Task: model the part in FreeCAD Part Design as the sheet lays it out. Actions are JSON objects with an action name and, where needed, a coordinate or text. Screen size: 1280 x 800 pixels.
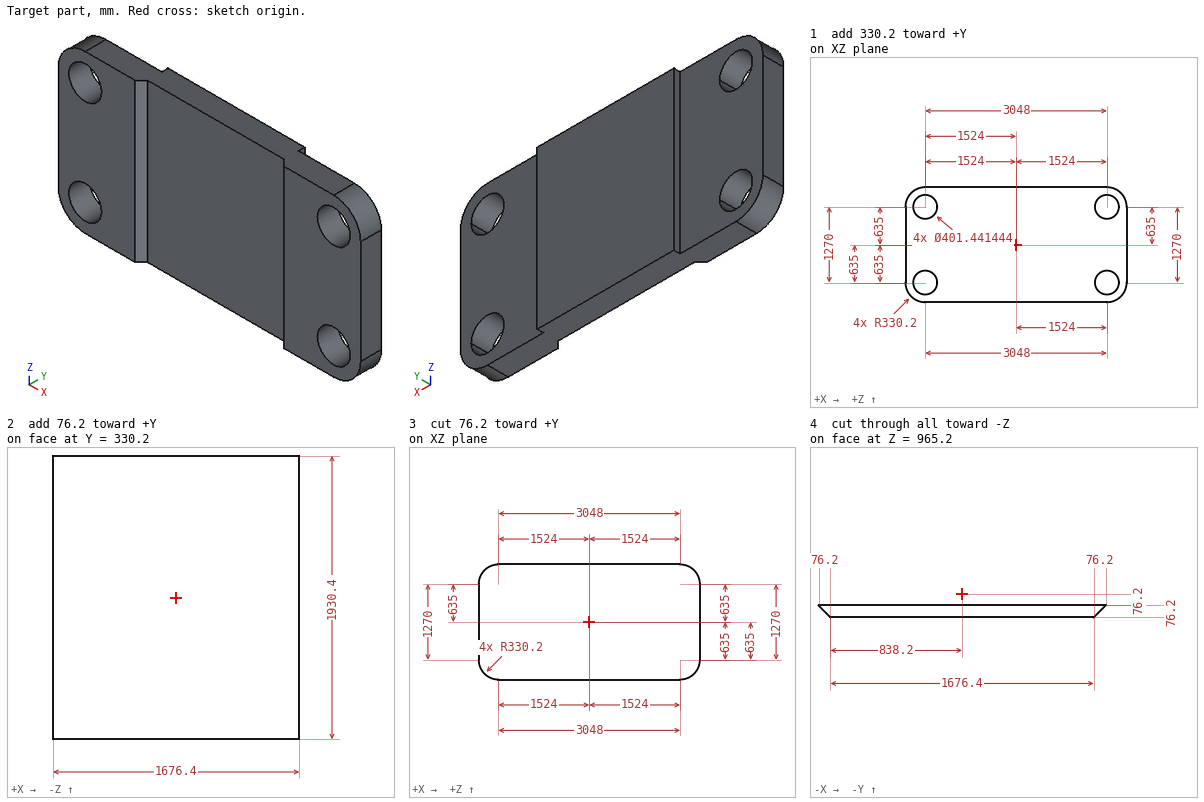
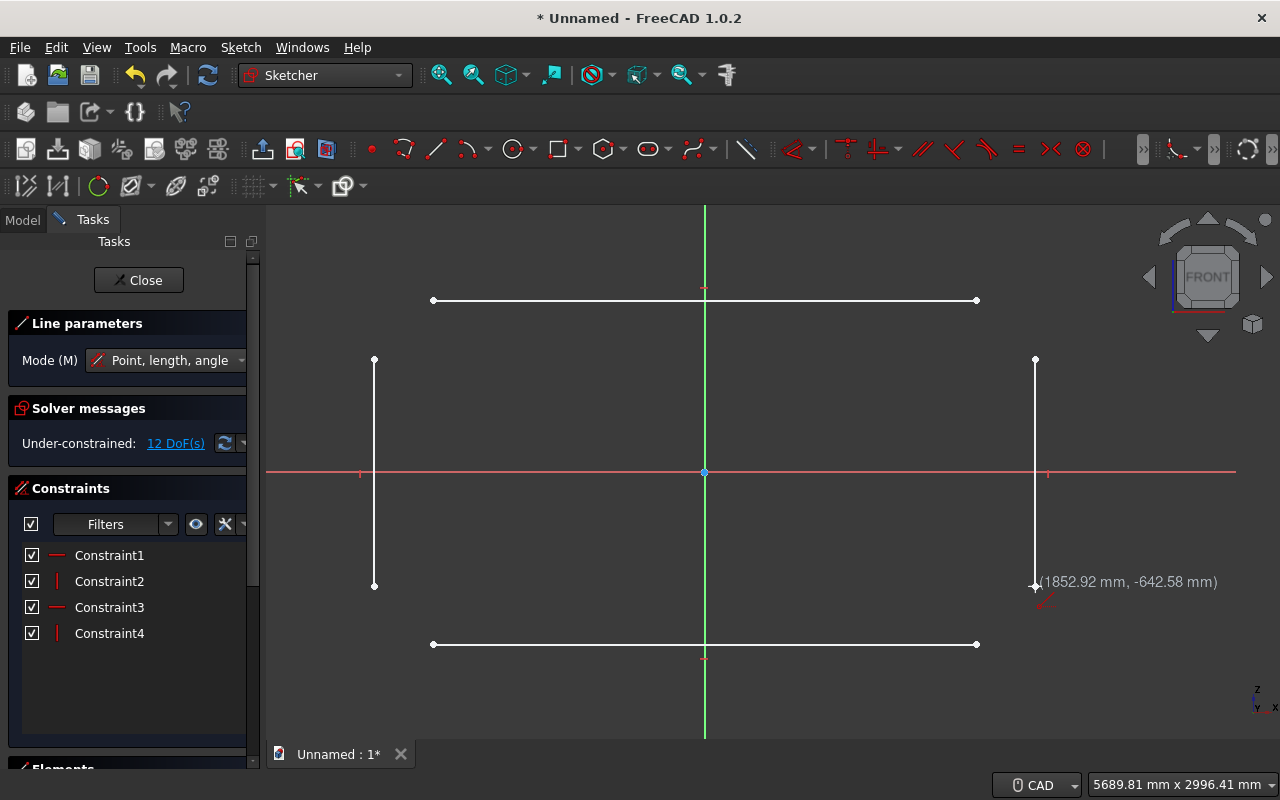
{"action": "key", "text": "g 3 a"}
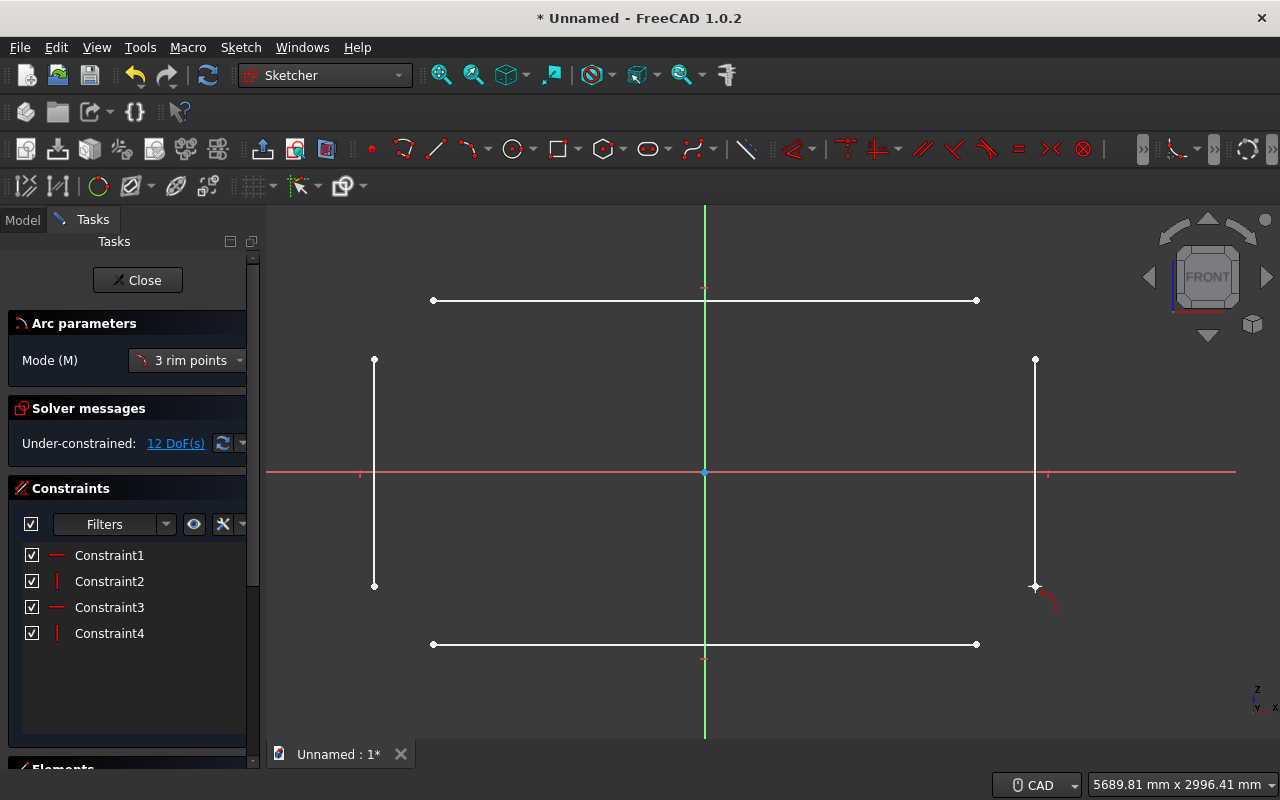
{"action": "left_click", "coordinate": [433, 645]}
{"action": "left_click", "coordinate": [374, 587]}
{"action": "left_click", "coordinate": [392, 627]}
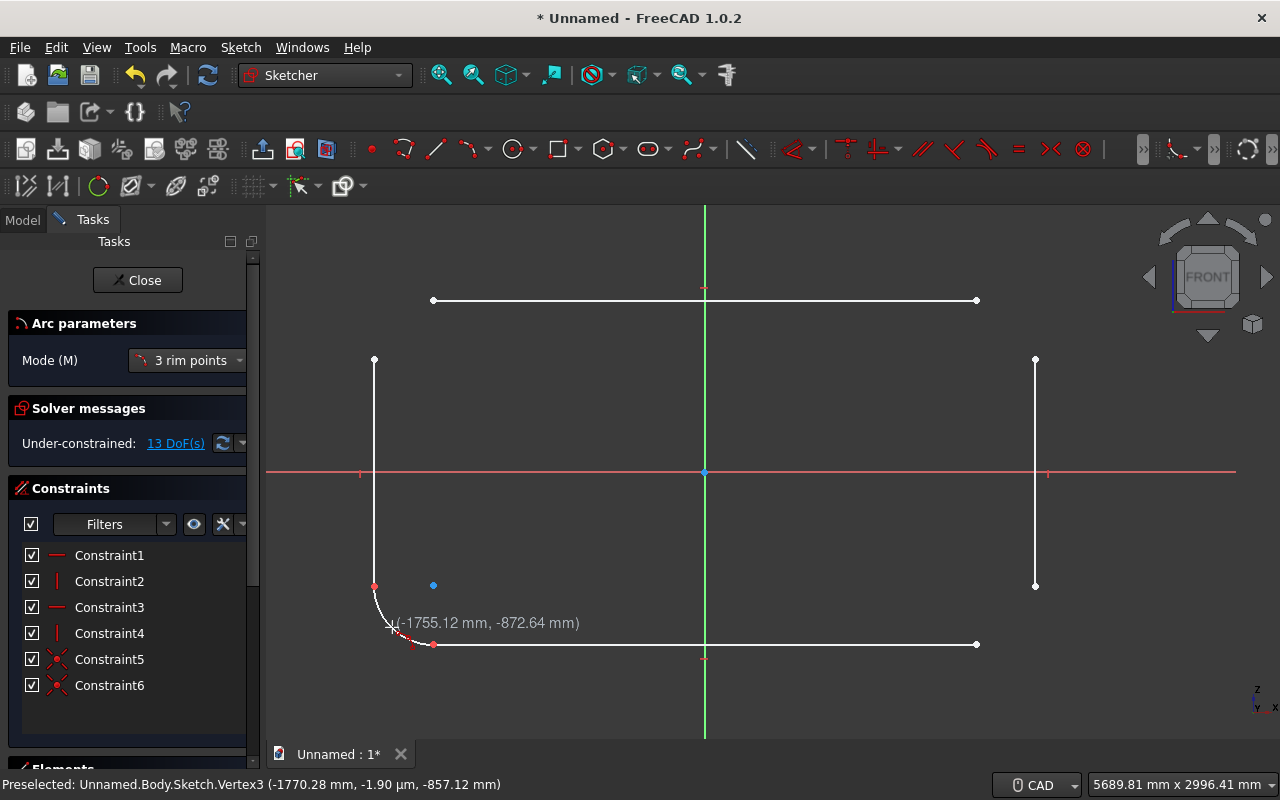
{"action": "left_click", "coordinate": [374, 360]}
{"action": "left_click", "coordinate": [433, 301]}
{"action": "left_click", "coordinate": [392, 318]}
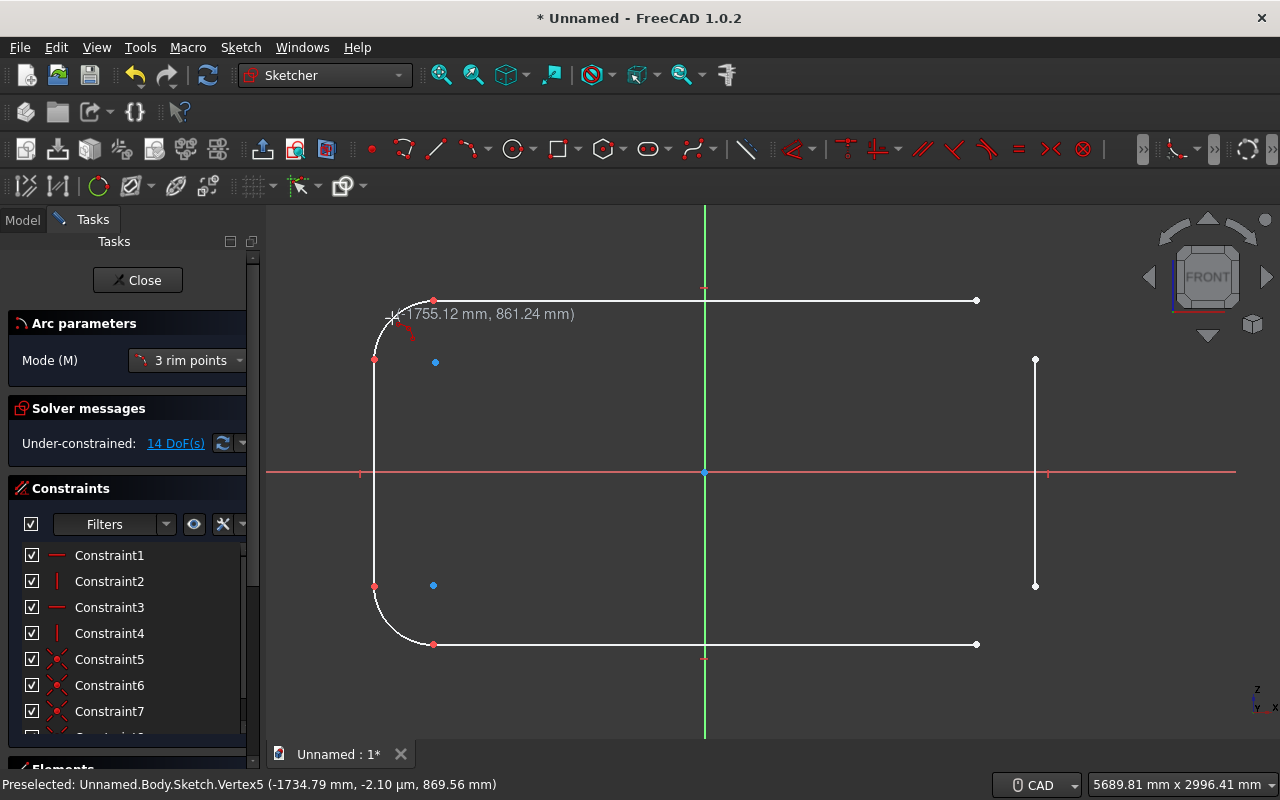
{"action": "left_click", "coordinate": [976, 301]}
{"action": "left_click", "coordinate": [1035, 360]}
{"action": "left_click", "coordinate": [1018, 318]}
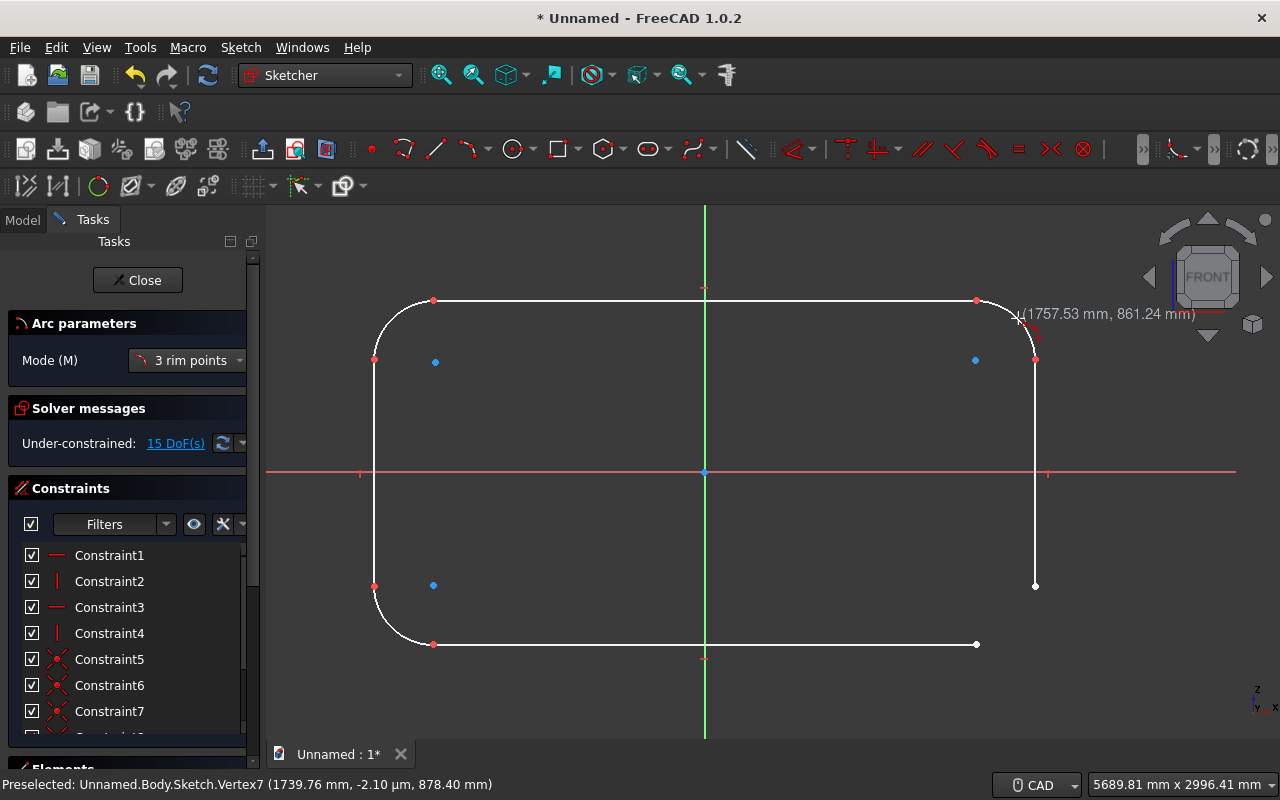
{"action": "left_click", "coordinate": [1035, 587]}
{"action": "left_click", "coordinate": [976, 645]}
{"action": "left_click", "coordinate": [1018, 627]}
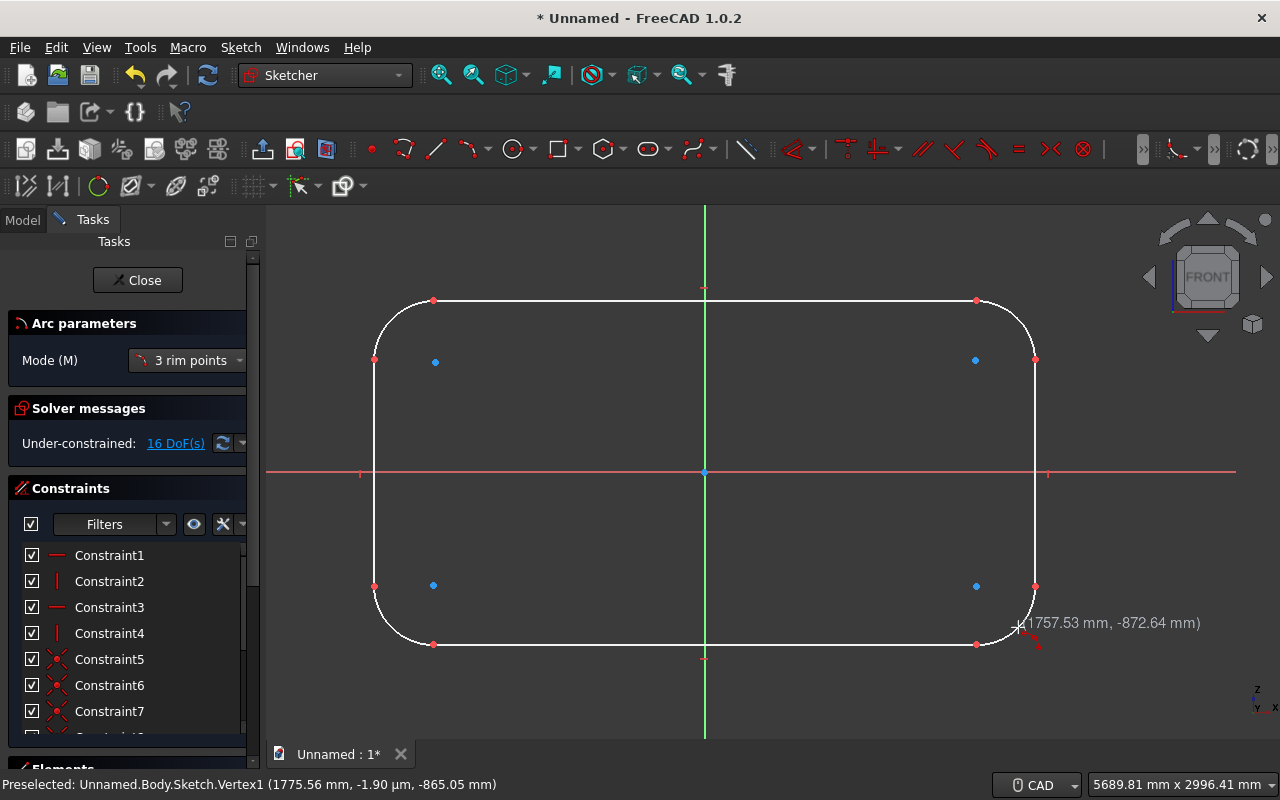
{"action": "key", "text": "g c"}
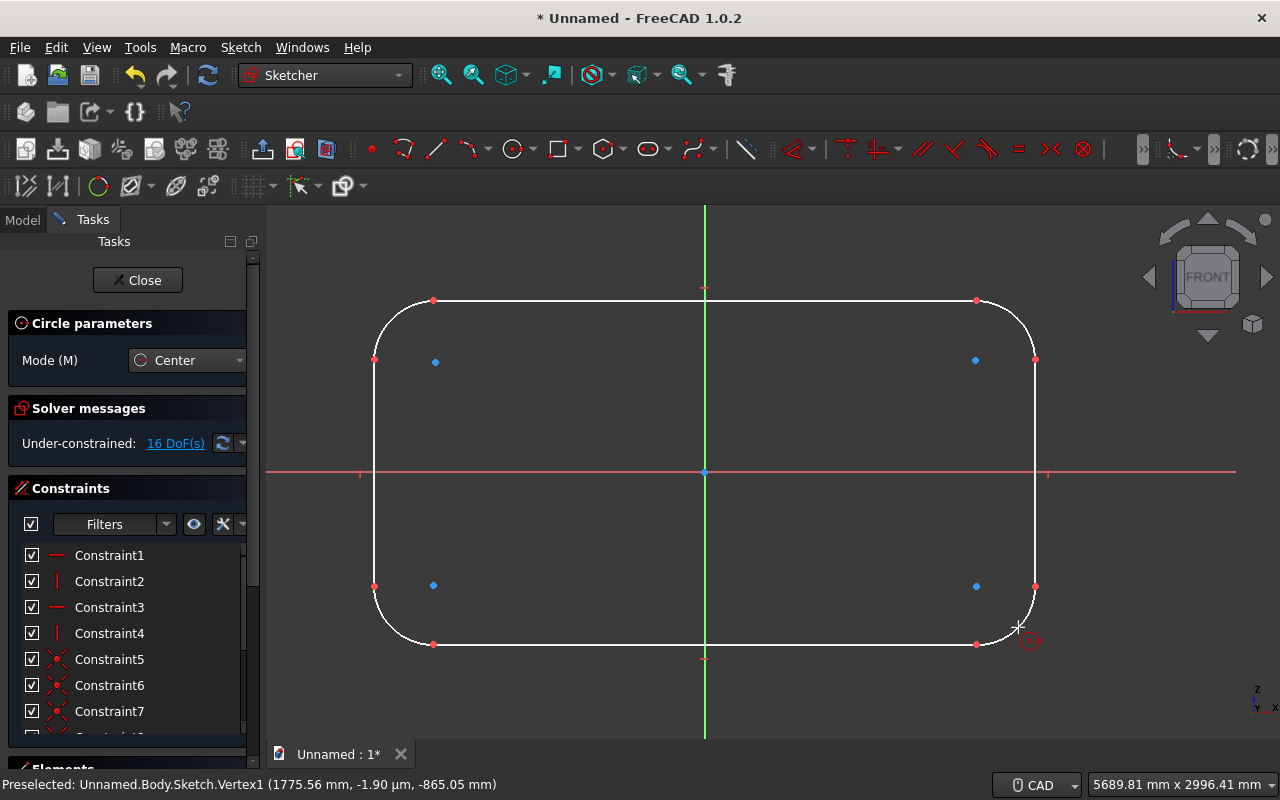
{"action": "left_click", "coordinate": [433, 359]}
{"action": "left_click", "coordinate": [458, 334]}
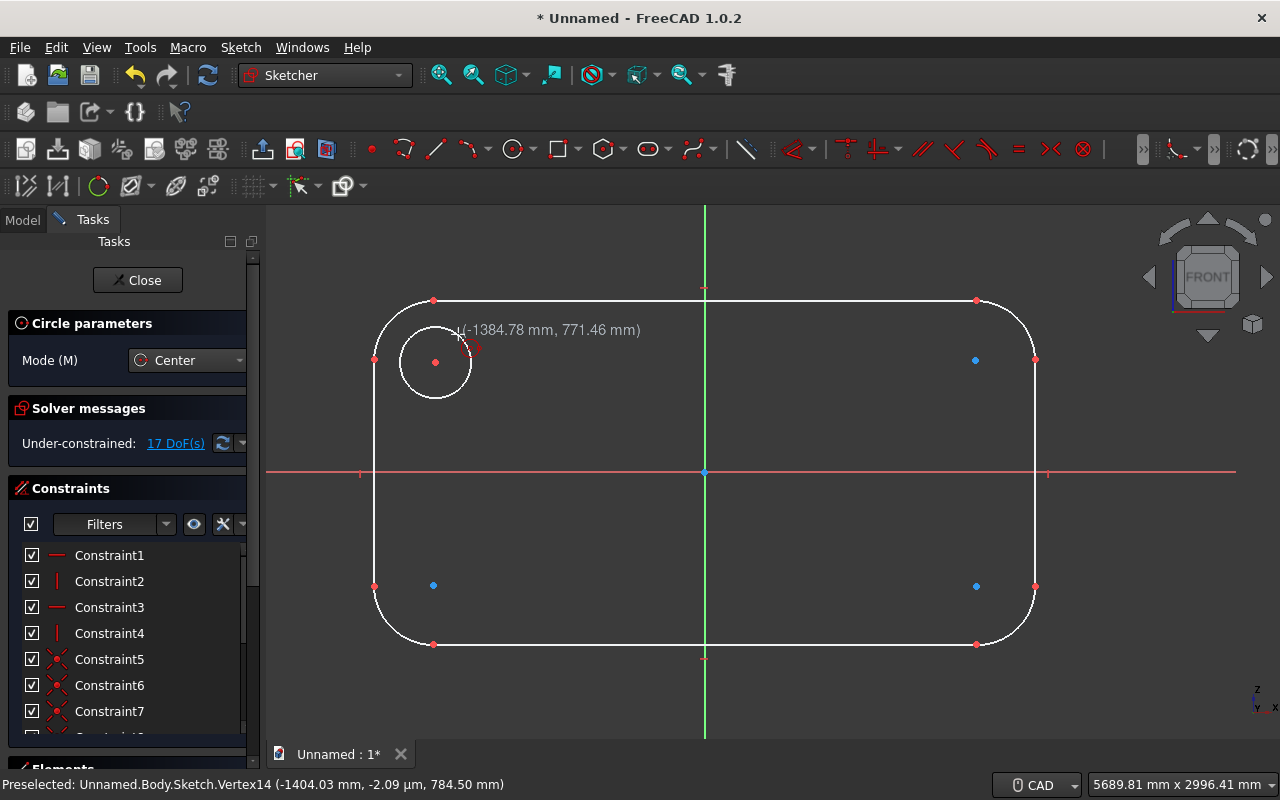
{"action": "left_click", "coordinate": [976, 359]}
{"action": "left_click", "coordinate": [1002, 334]}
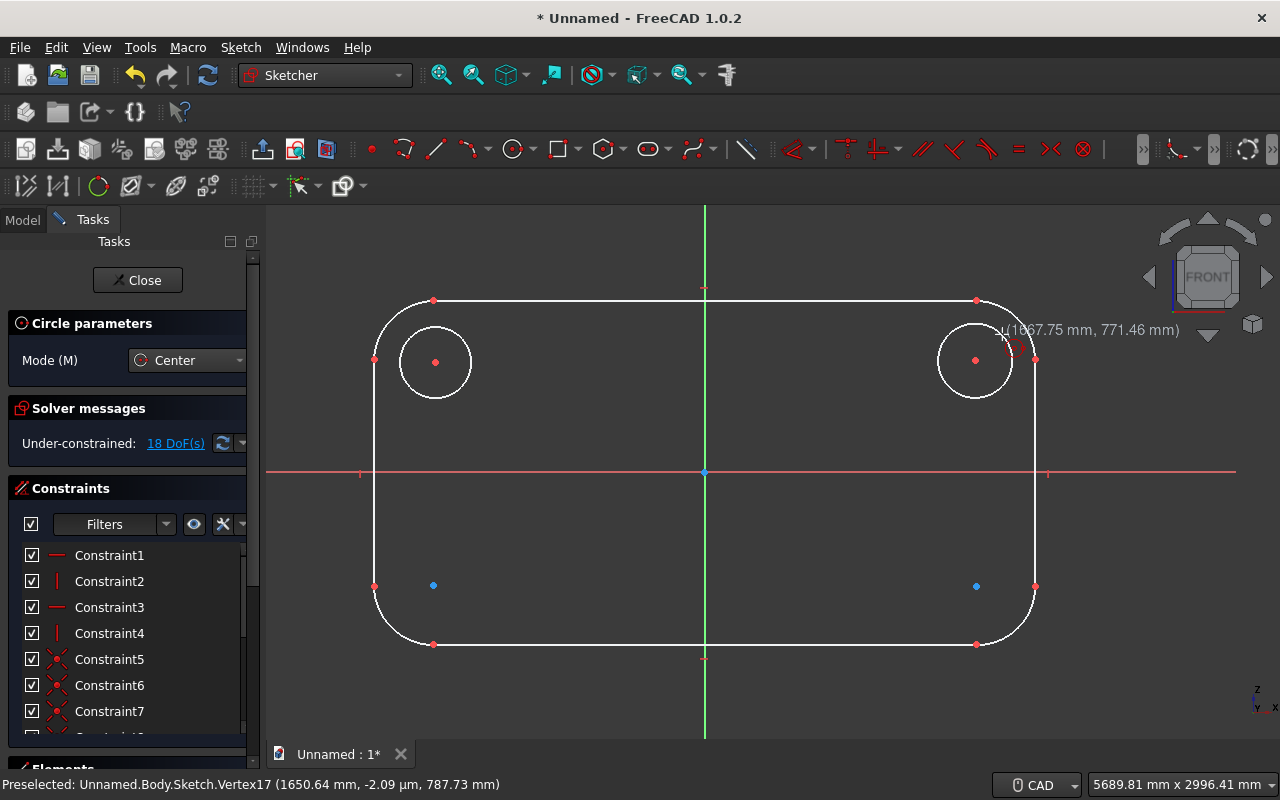
{"action": "left_click", "coordinate": [433, 586]}
{"action": "left_click", "coordinate": [458, 560]}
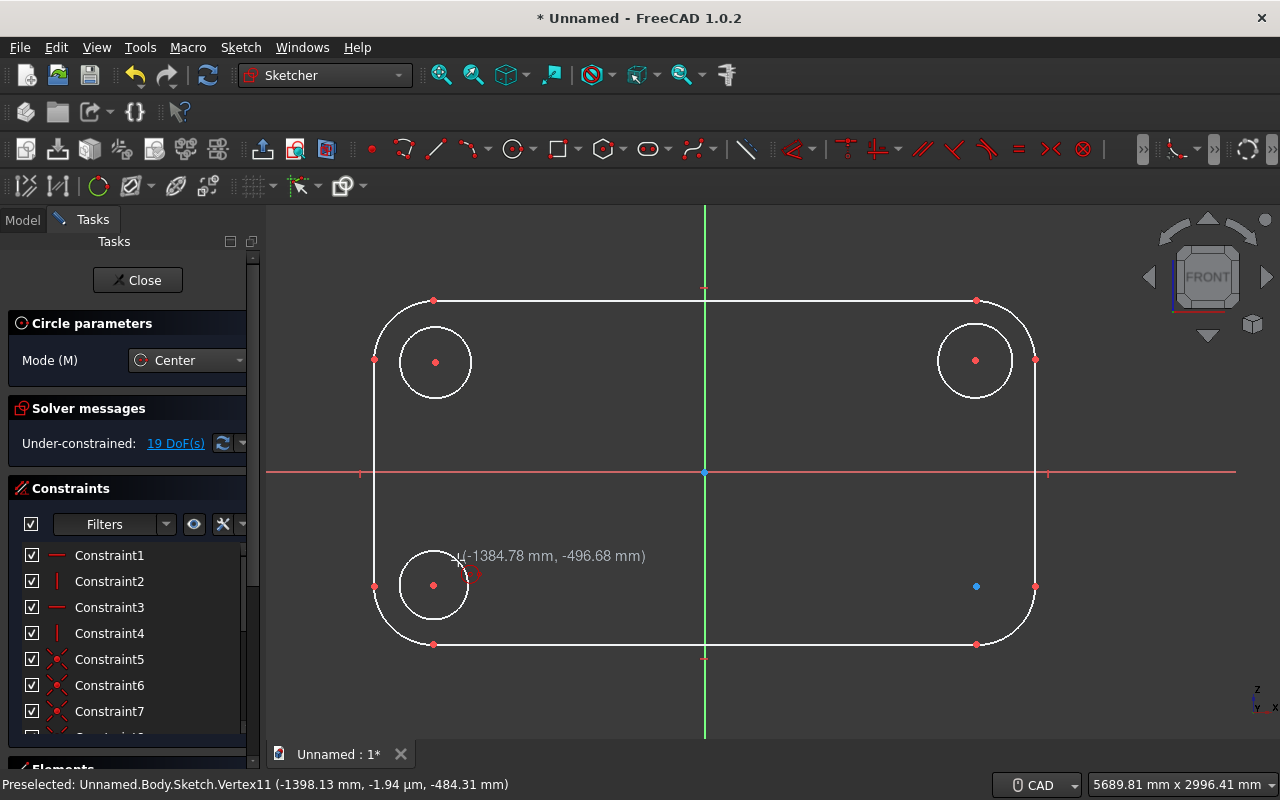
{"action": "left_click", "coordinate": [976, 586]}
{"action": "left_click", "coordinate": [1002, 560]}
{"action": "key", "text": "Escape"}